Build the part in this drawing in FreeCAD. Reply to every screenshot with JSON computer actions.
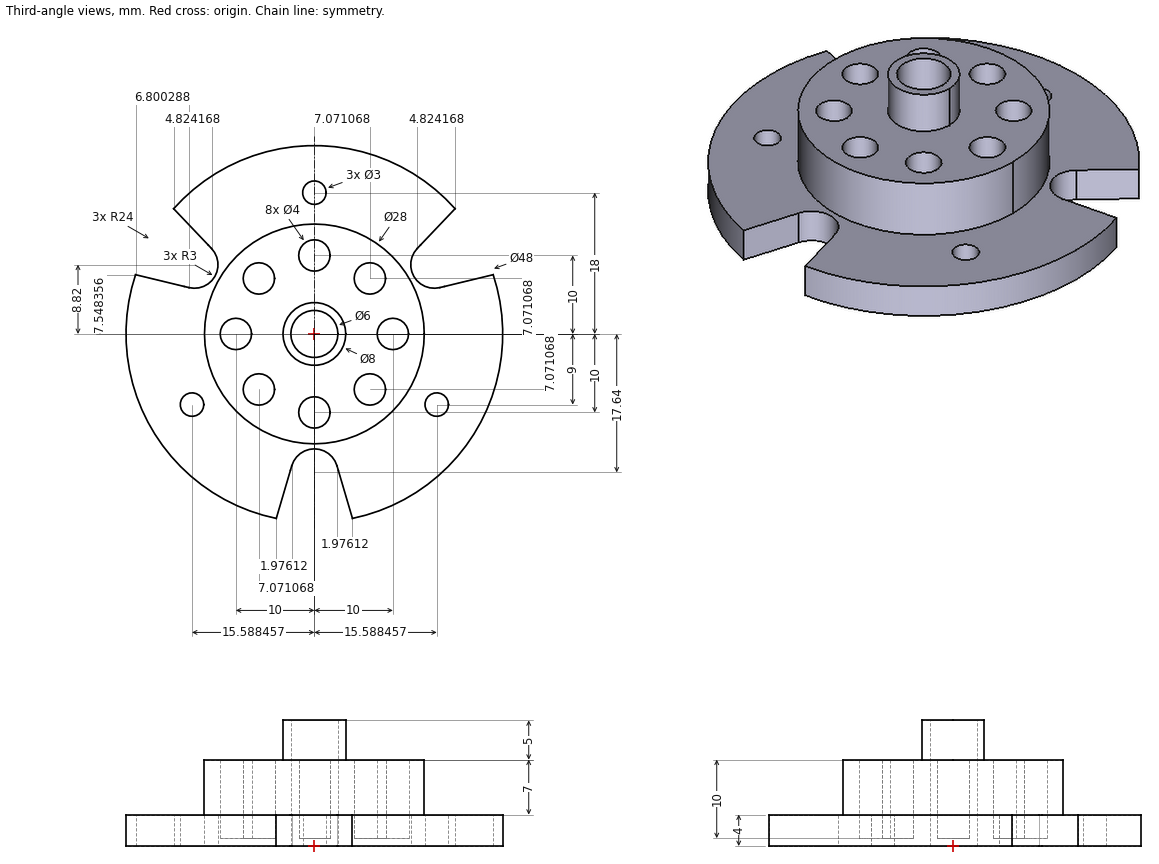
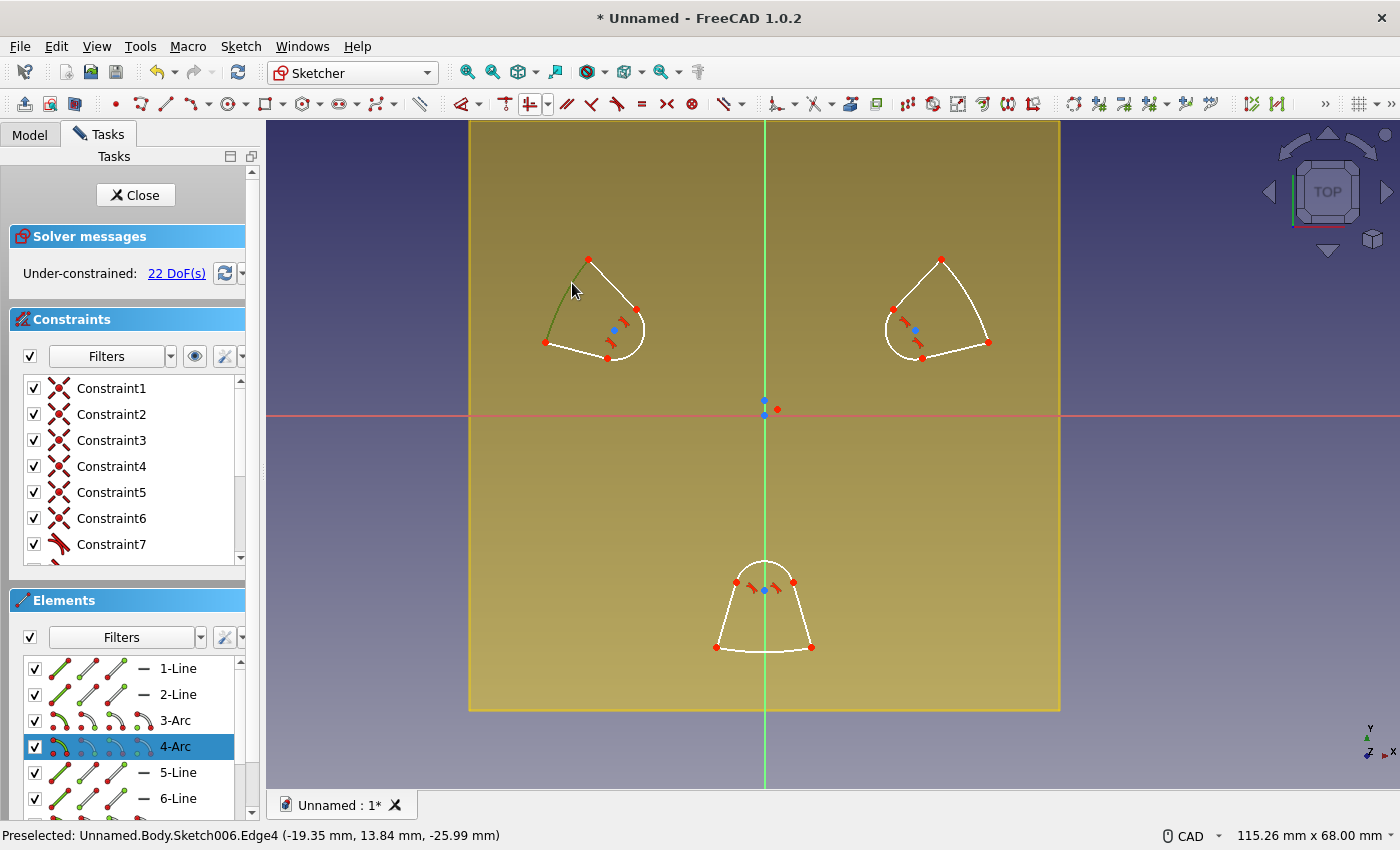
{"action": "left_click", "coordinate": [745, 652]}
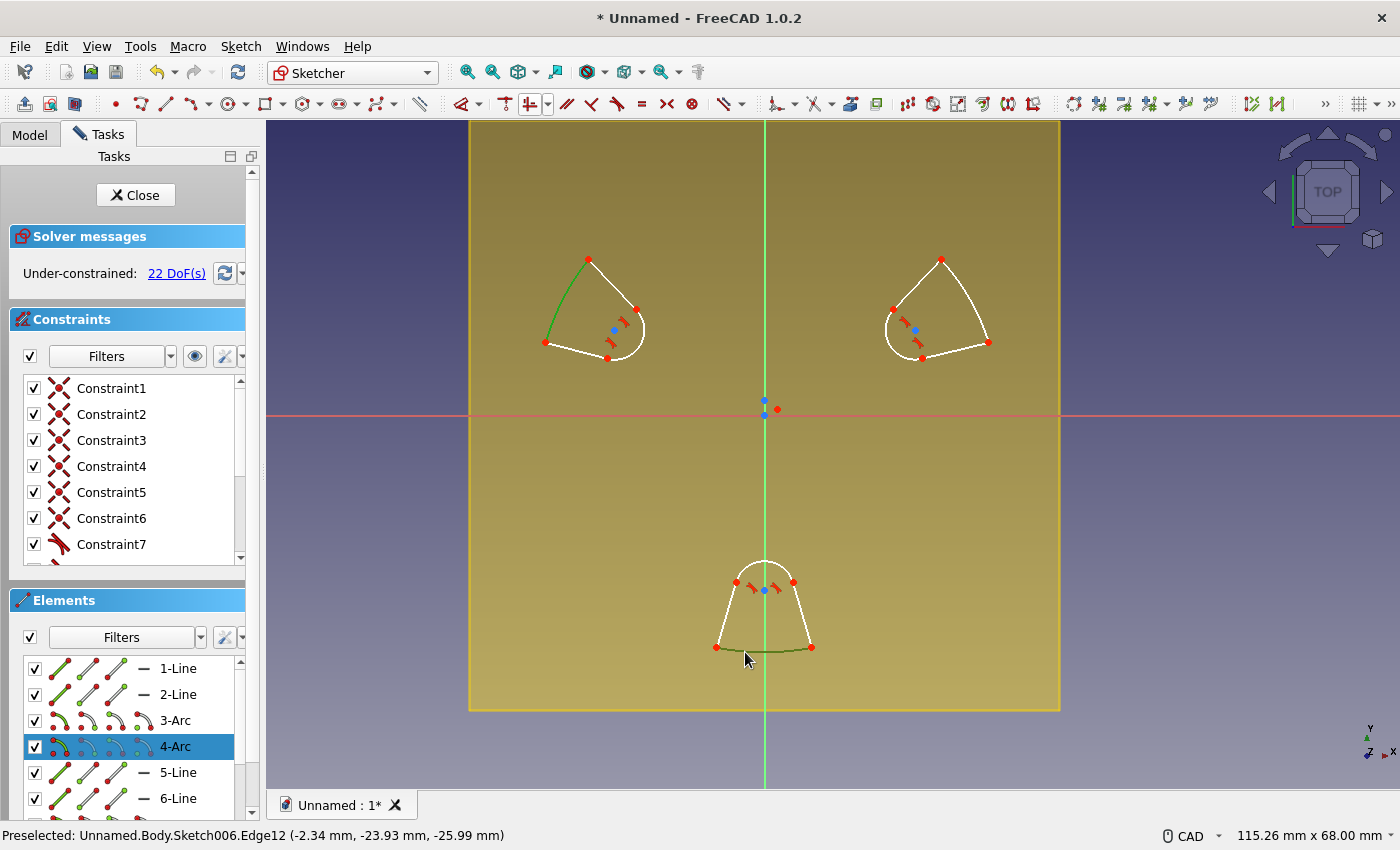
{"action": "key", "text": "c"}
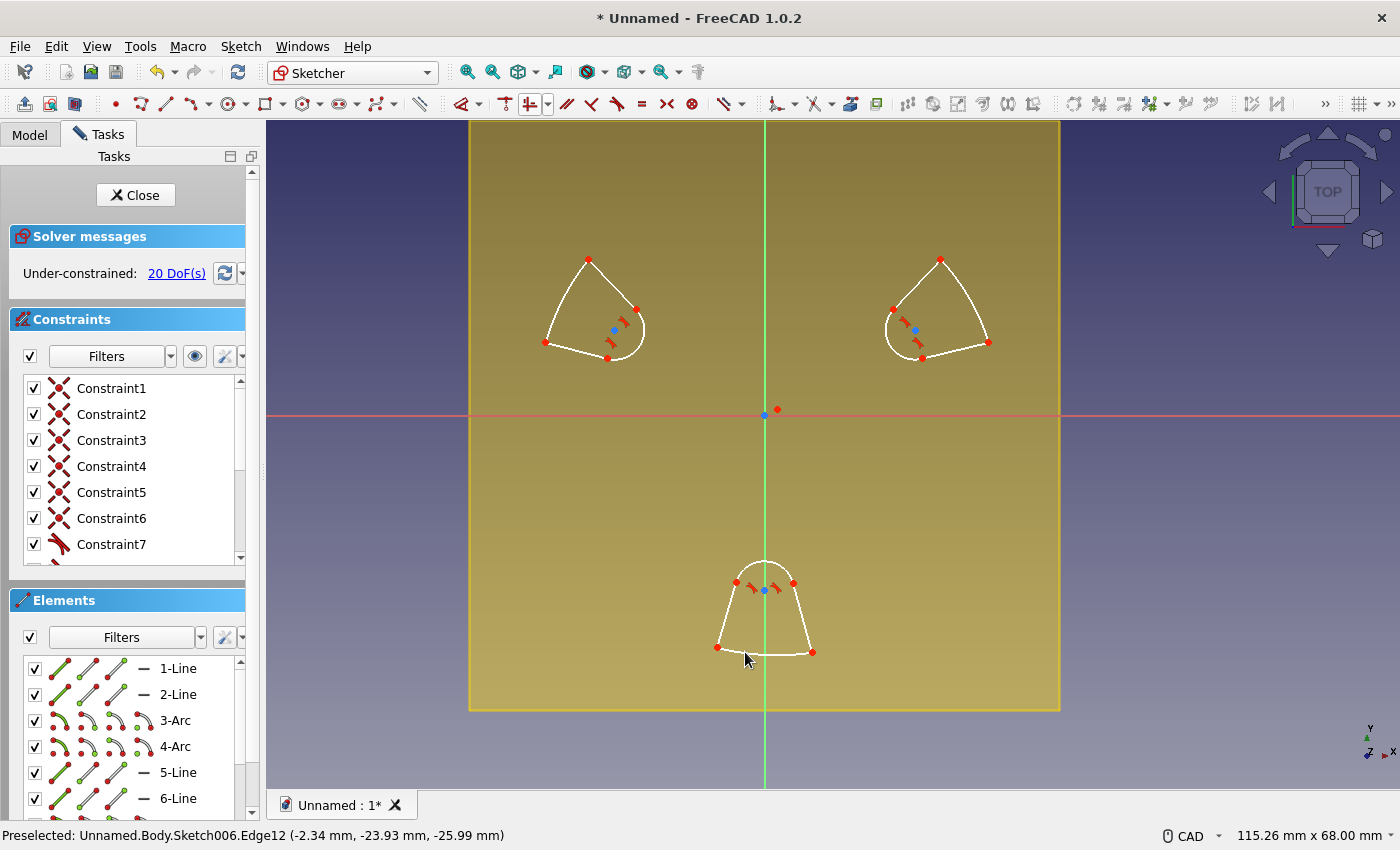
{"action": "scroll", "coordinate": [771, 413], "scroll_direction": "up", "scroll_amount": 2}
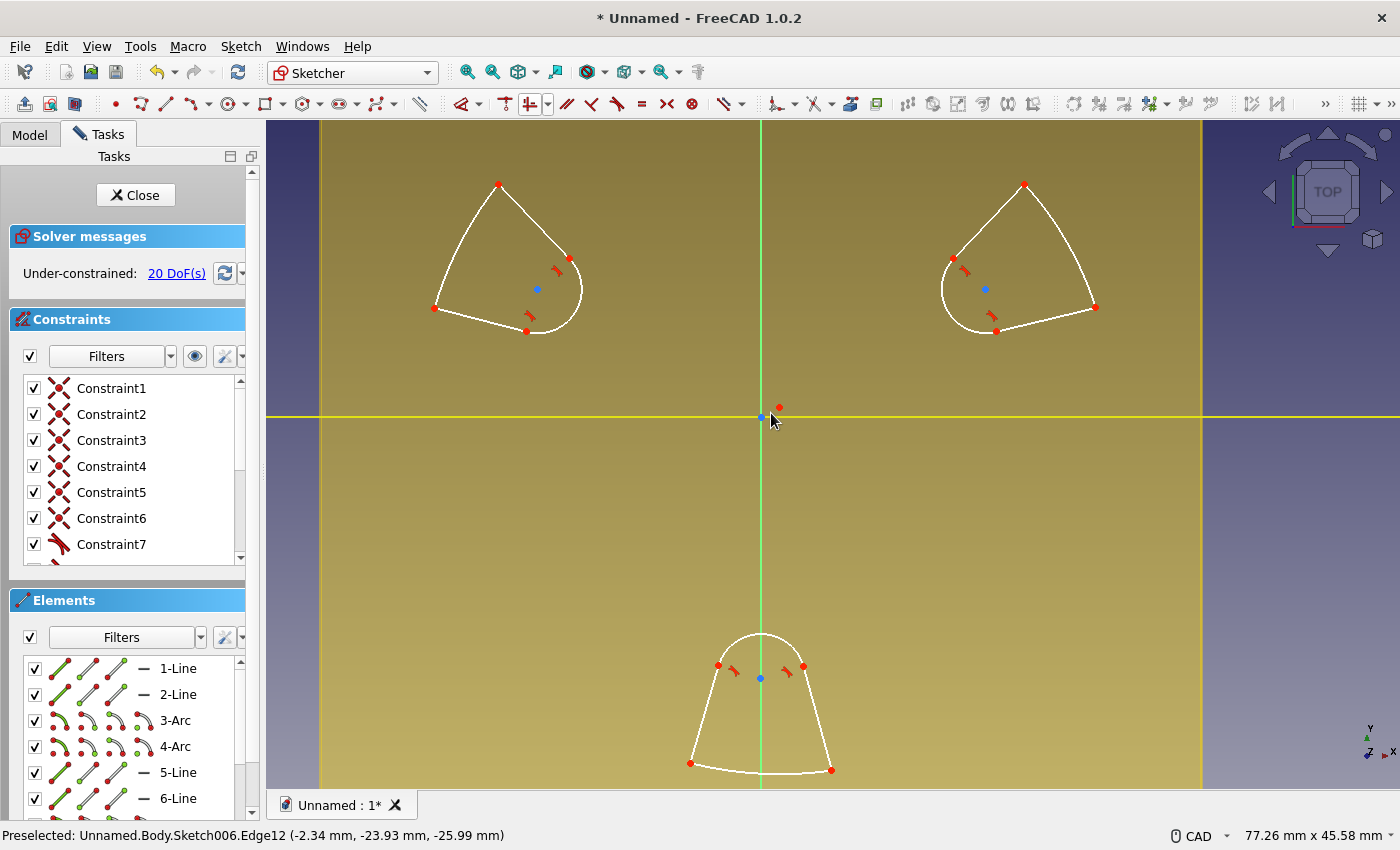
{"action": "left_click_drag", "start_coordinate": [751, 398], "coordinate": [790, 427]}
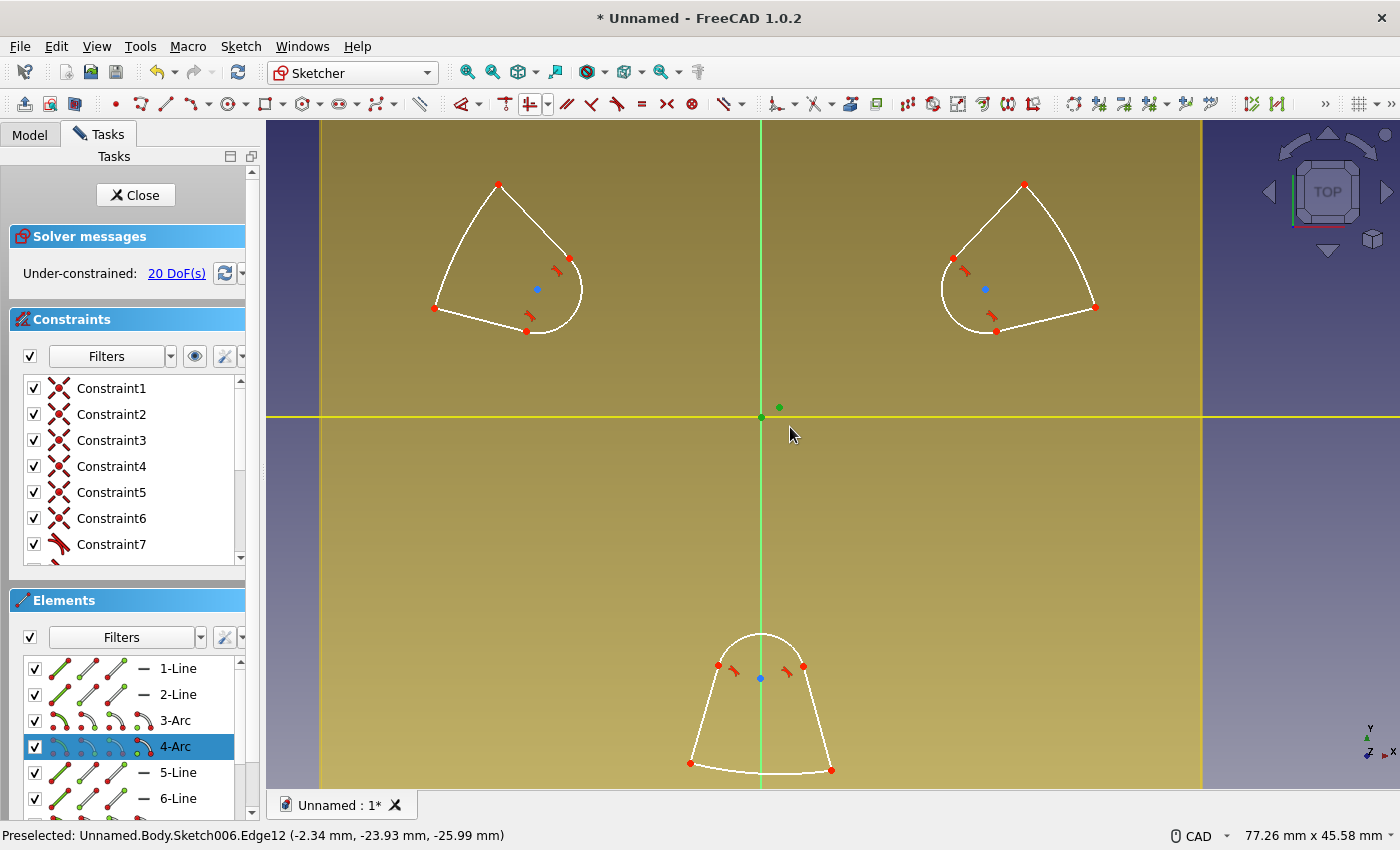
{"action": "left_click", "coordinate": [505, 104]}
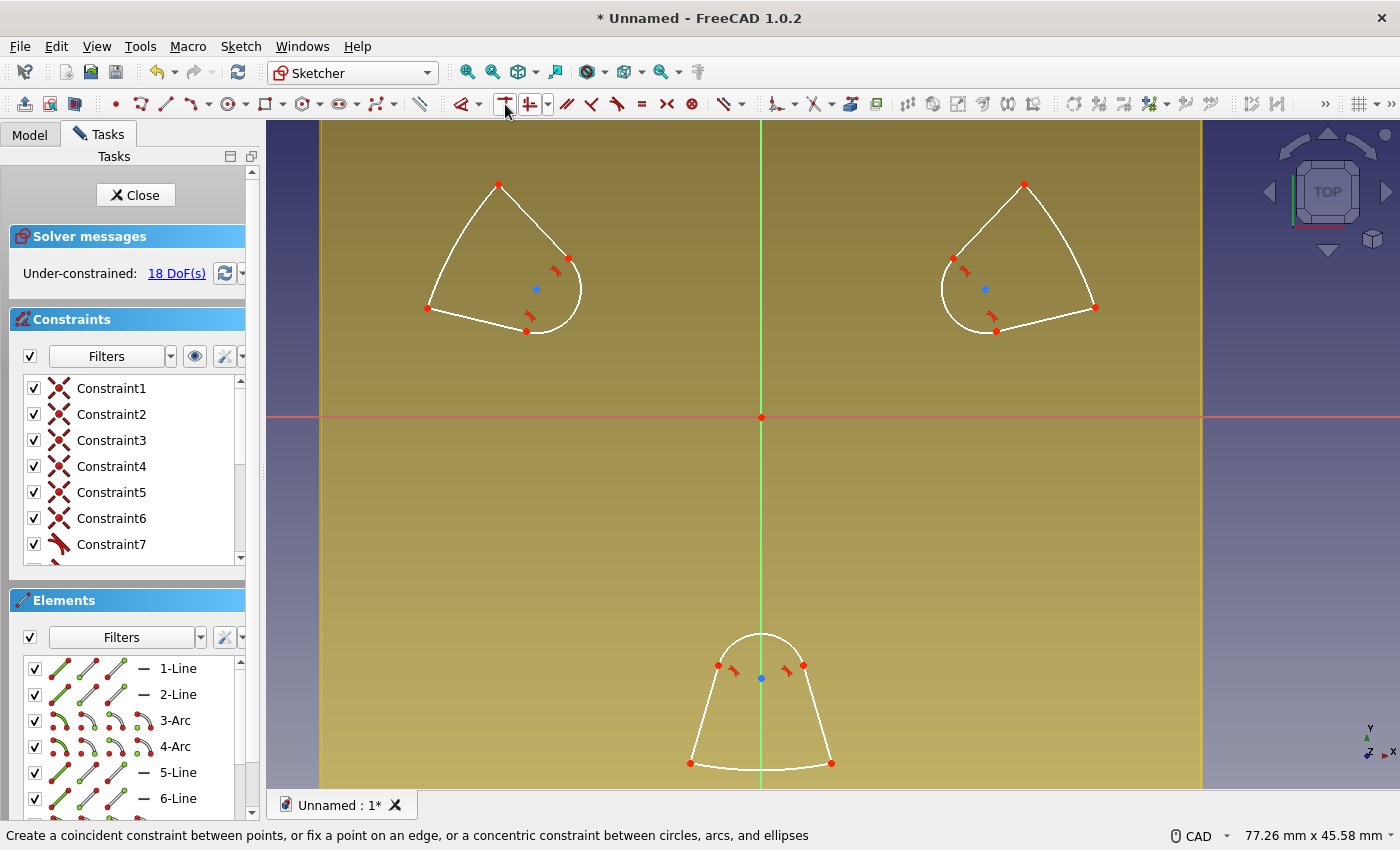
{"action": "left_click", "coordinate": [559, 327]}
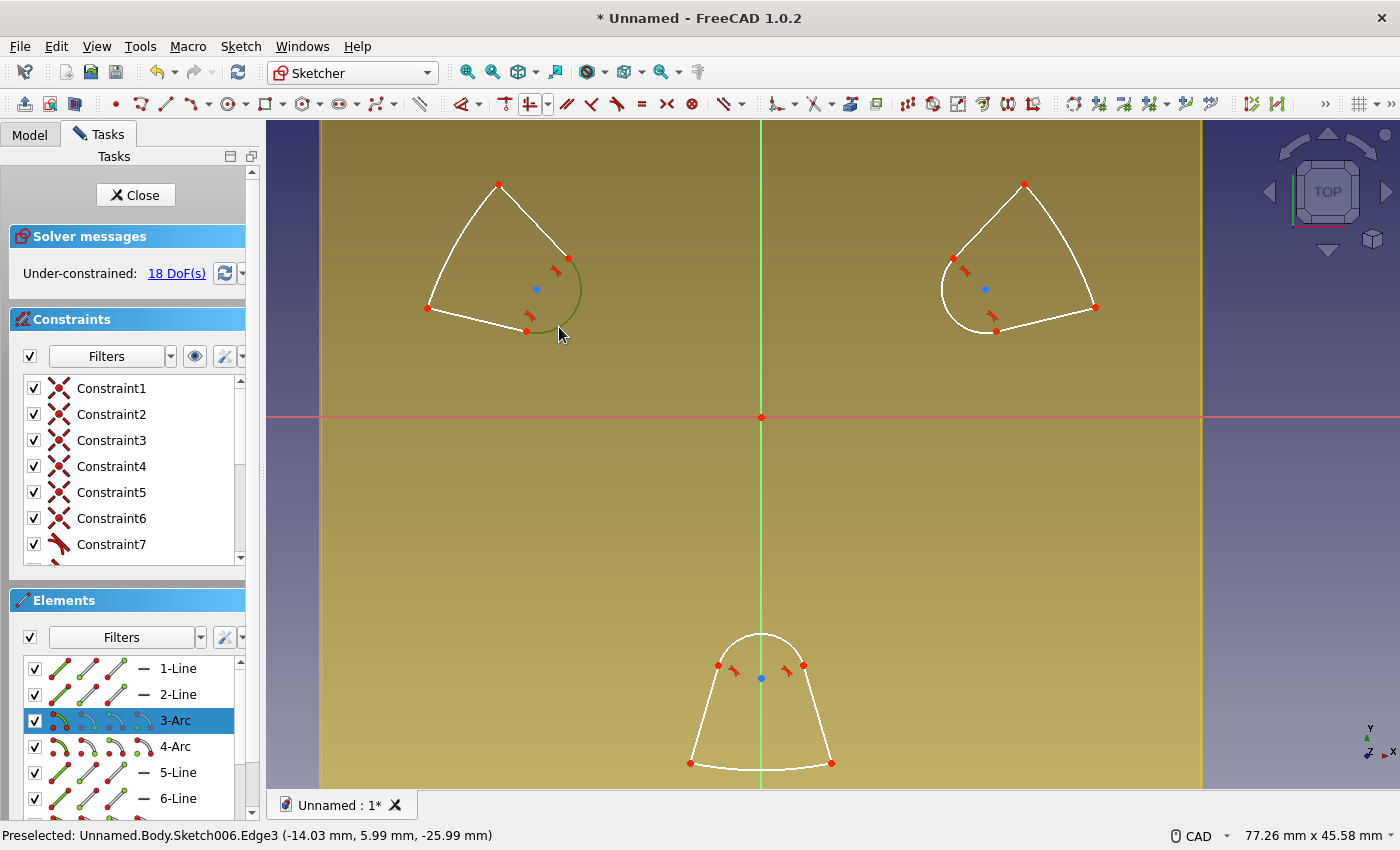
{"action": "left_click", "coordinate": [942, 290]}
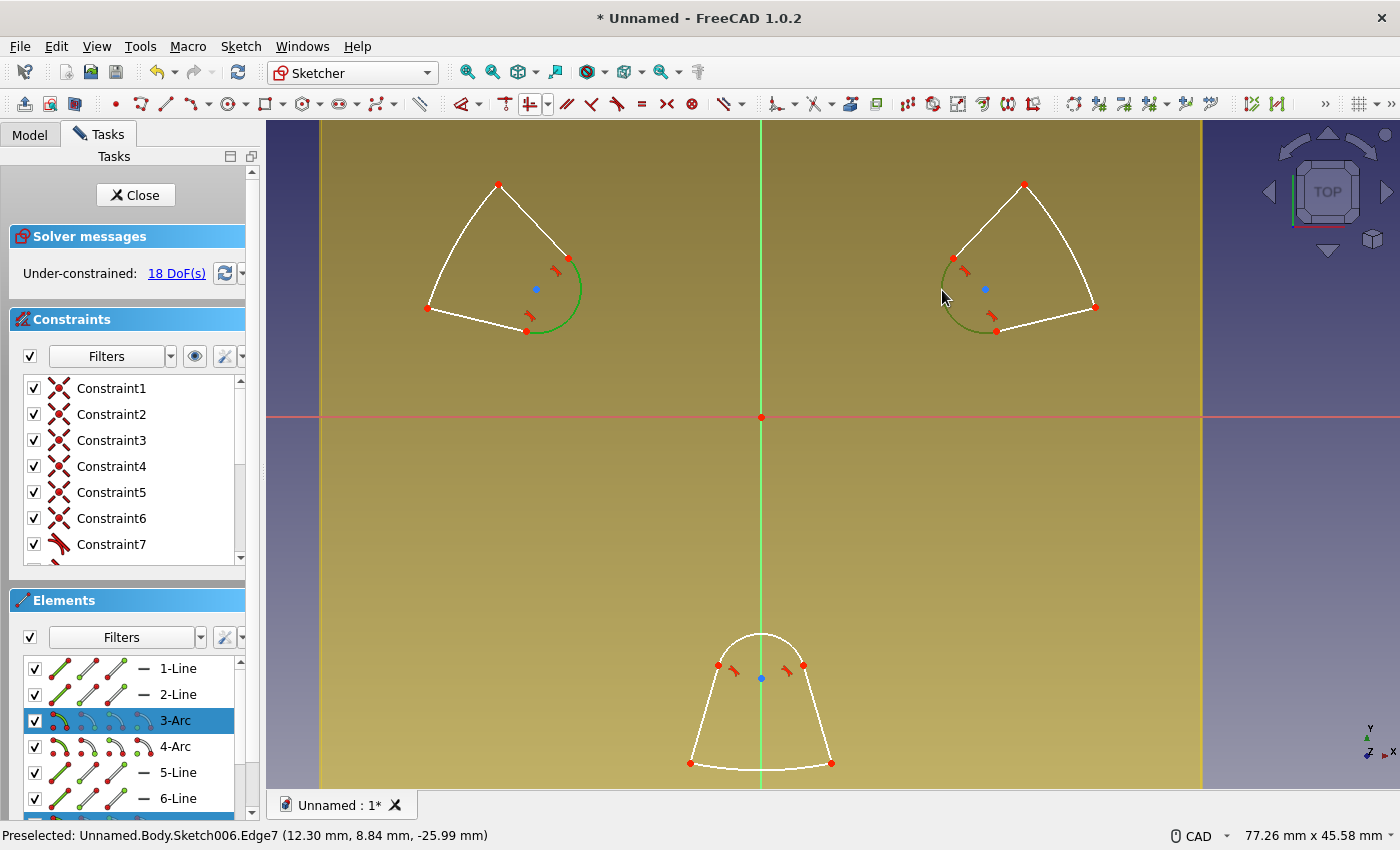
{"action": "left_click", "coordinate": [783, 640]}